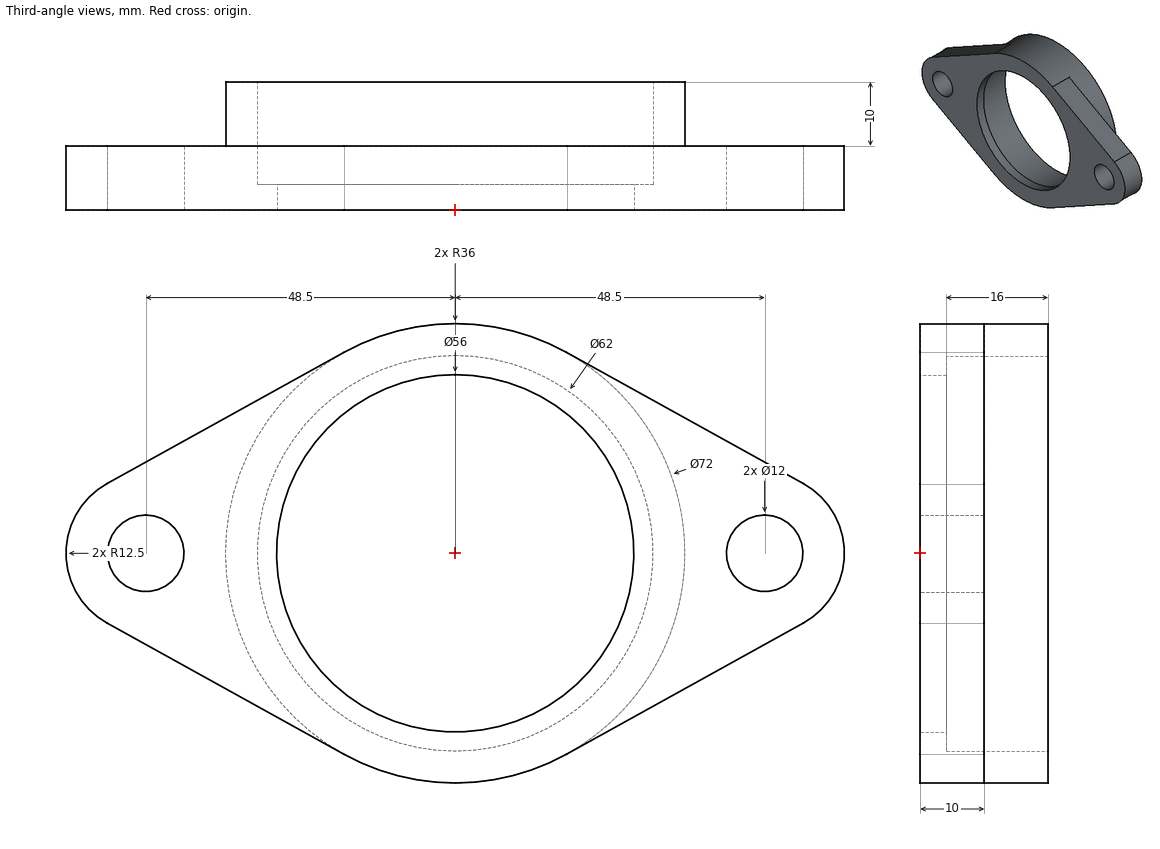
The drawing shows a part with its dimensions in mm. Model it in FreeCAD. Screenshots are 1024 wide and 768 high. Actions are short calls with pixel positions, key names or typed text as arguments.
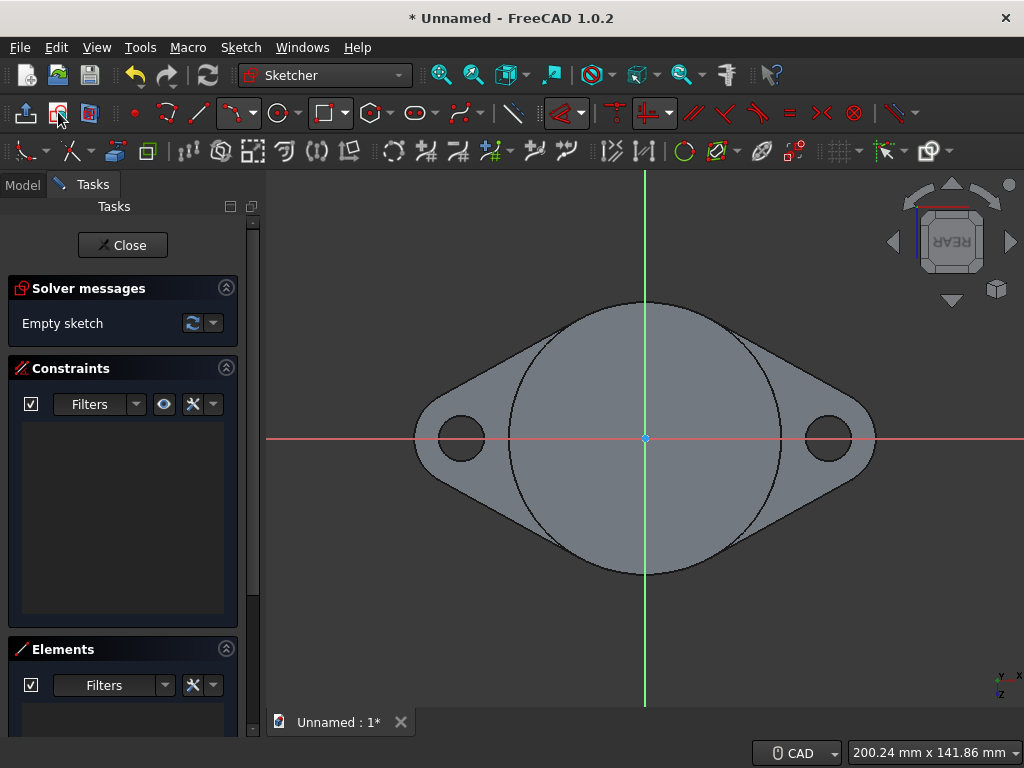
scroll(784, 438, up, 2)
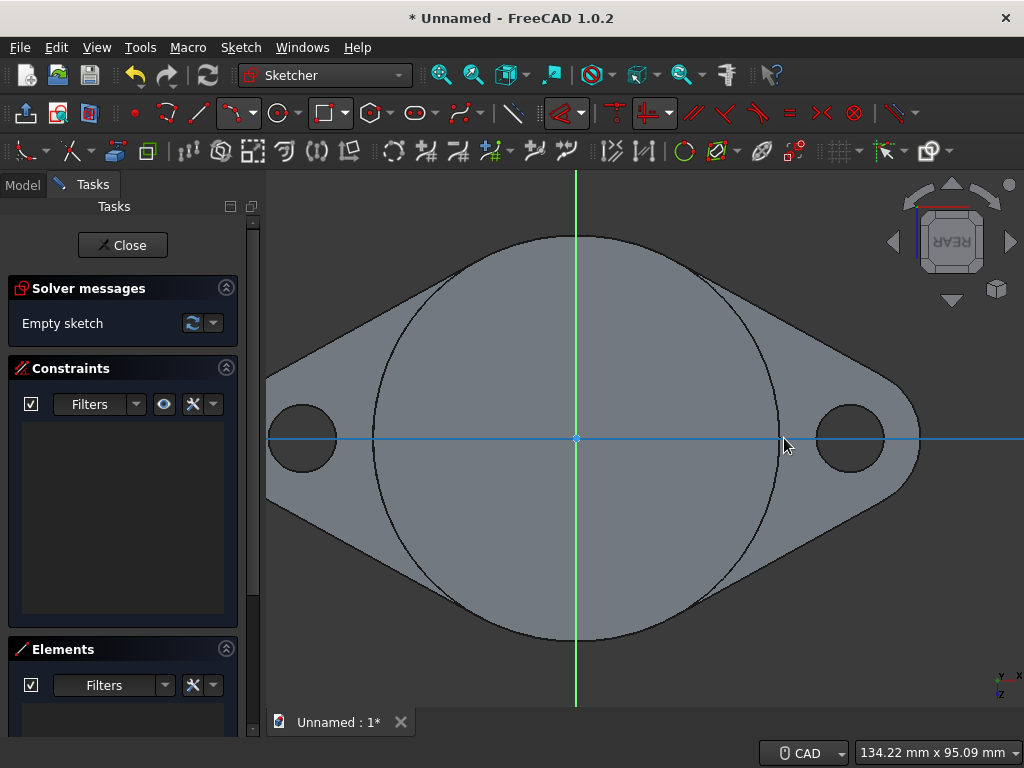
click(278, 114)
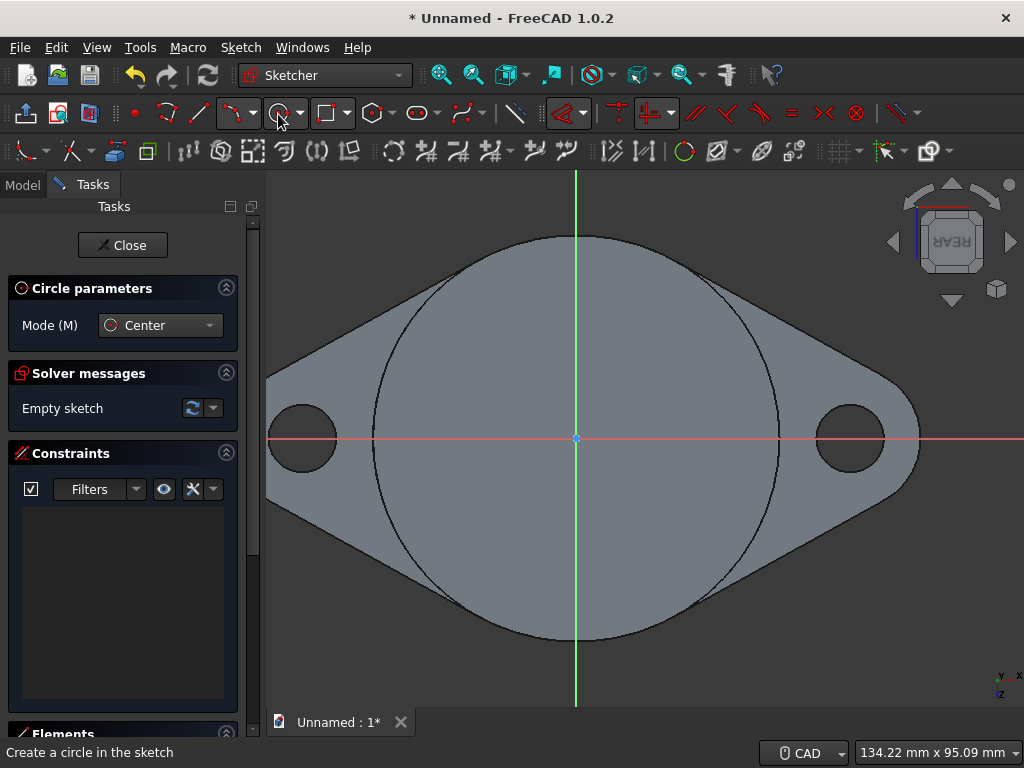
click(576, 438)
click(700, 315)
key(Escape)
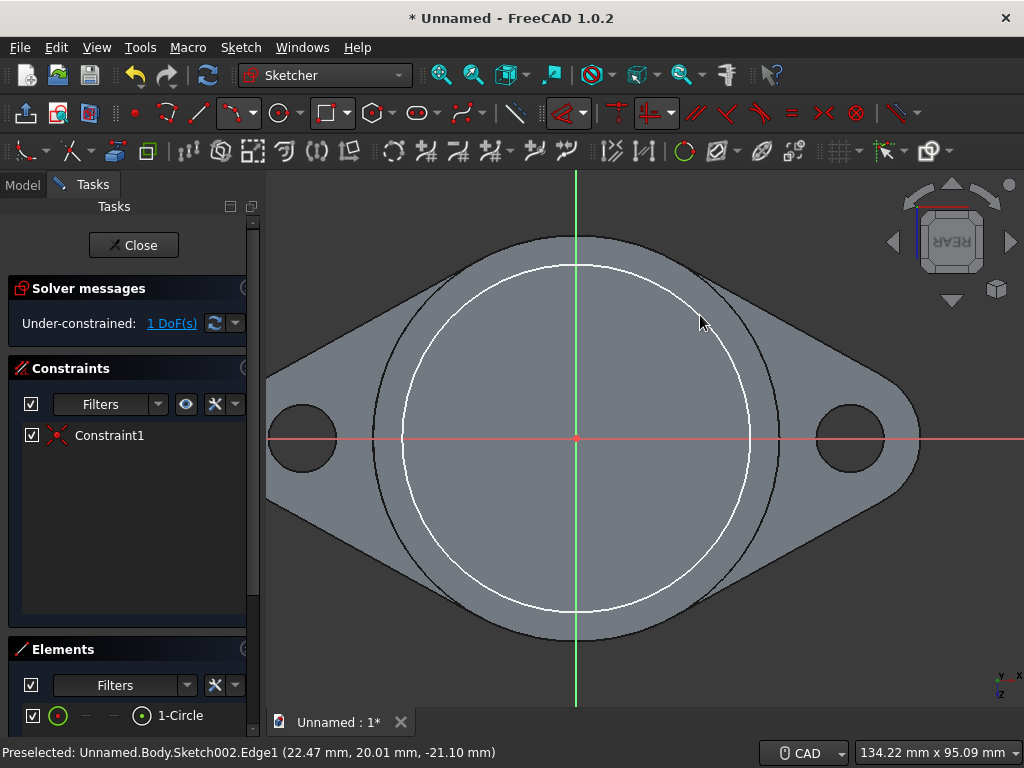
click(699, 315)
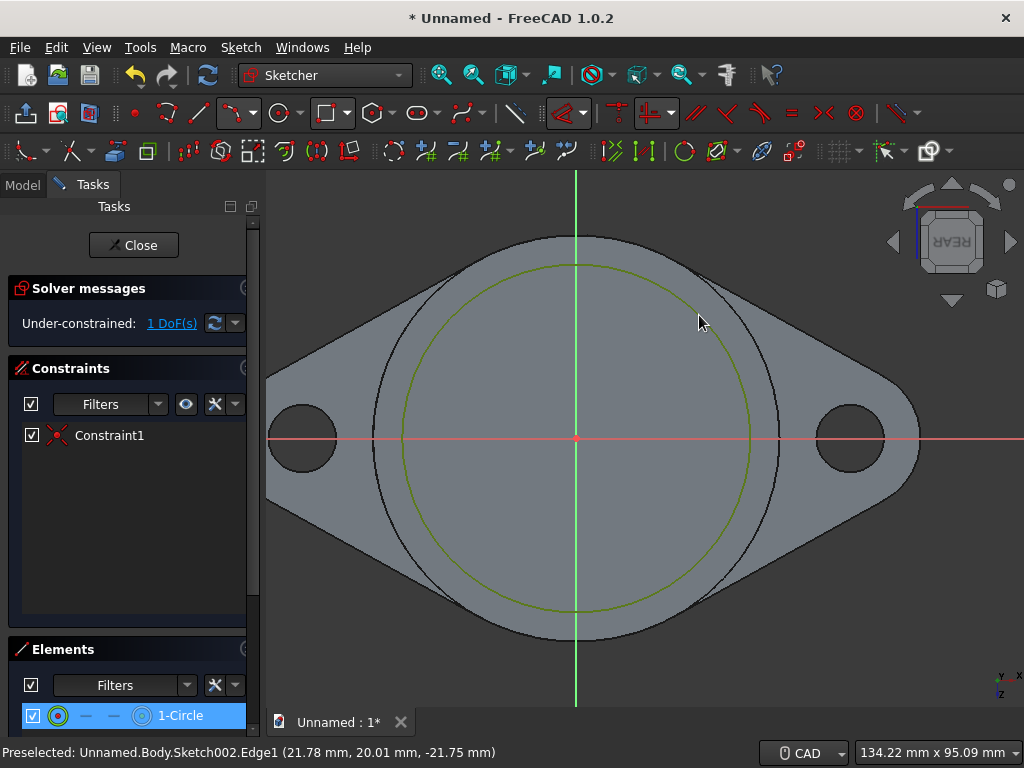
key(k)
key(o)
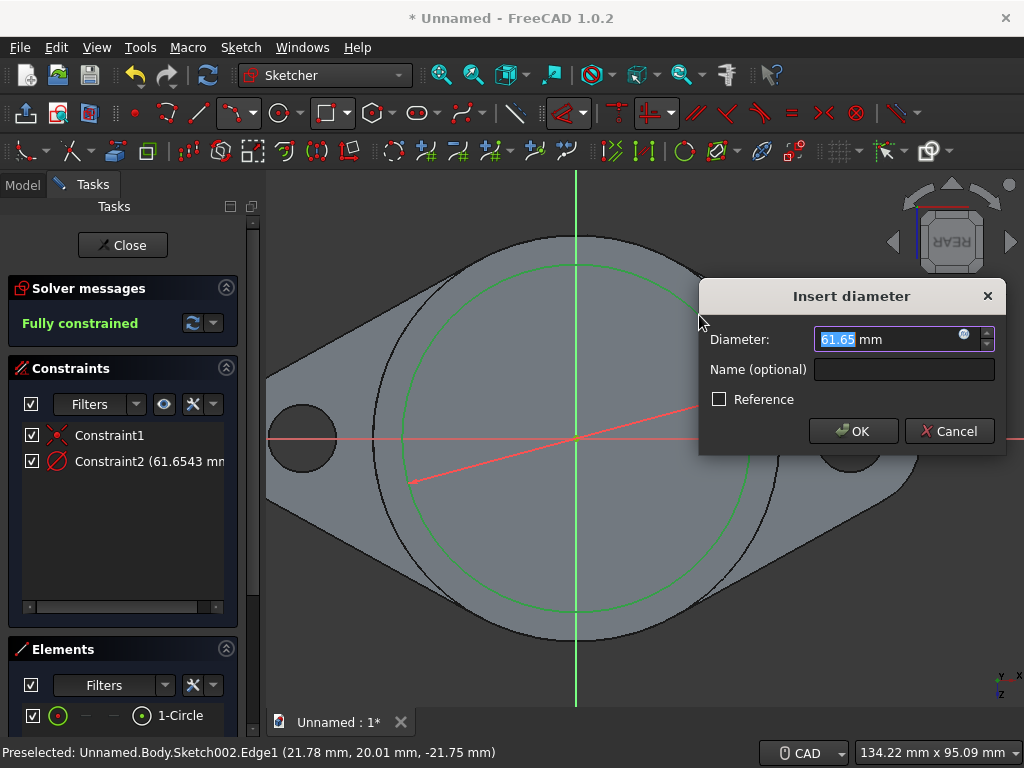
text(62)
key(Return)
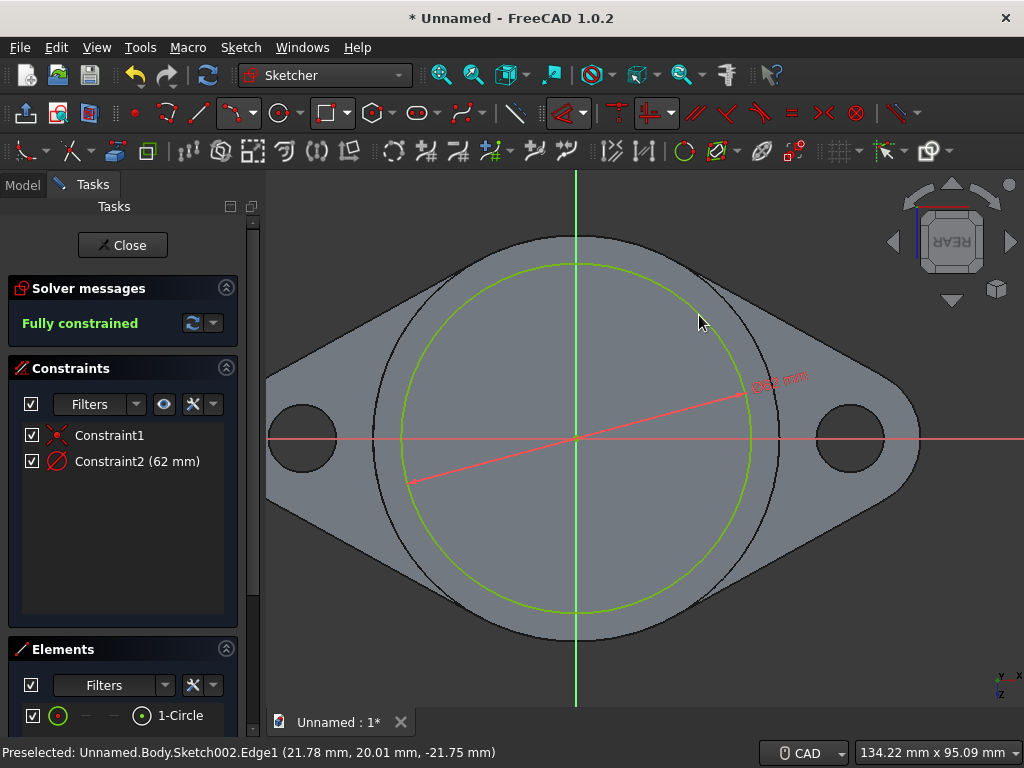
click(123, 245)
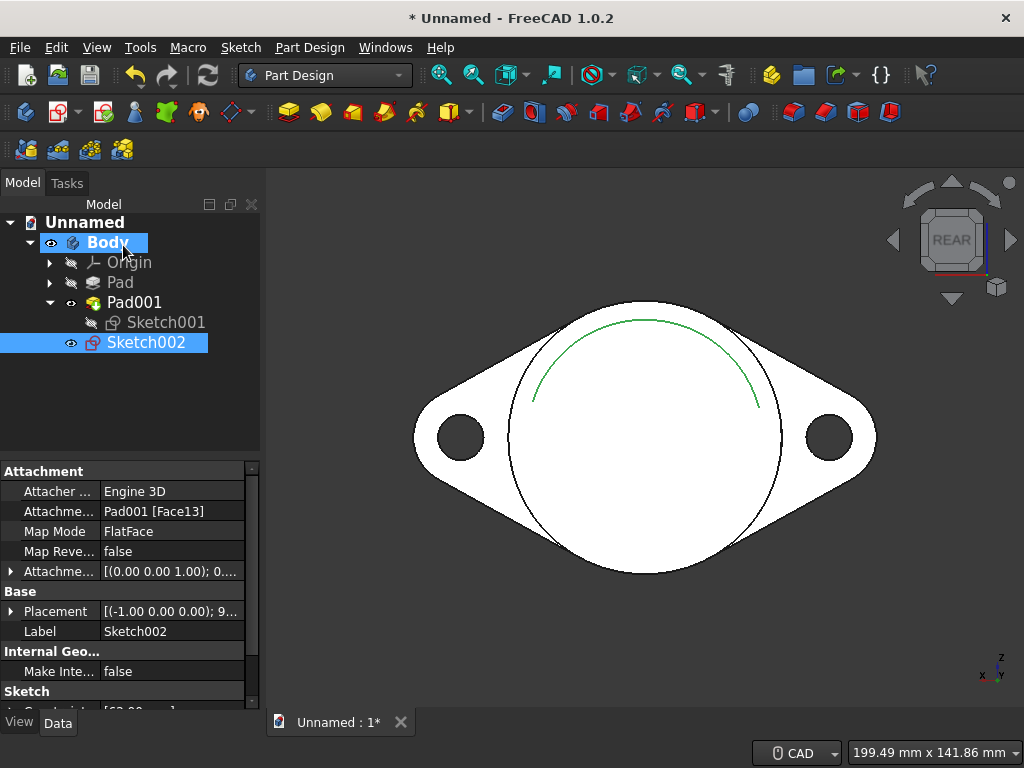
click(504, 112)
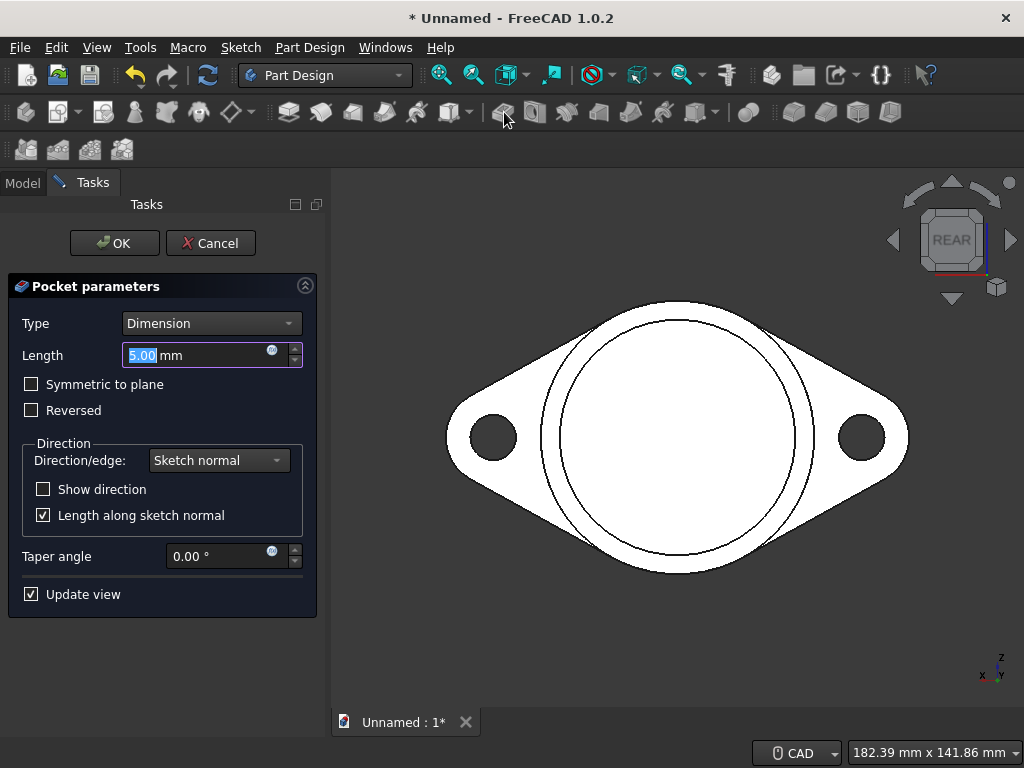
text(16)
key(Tab)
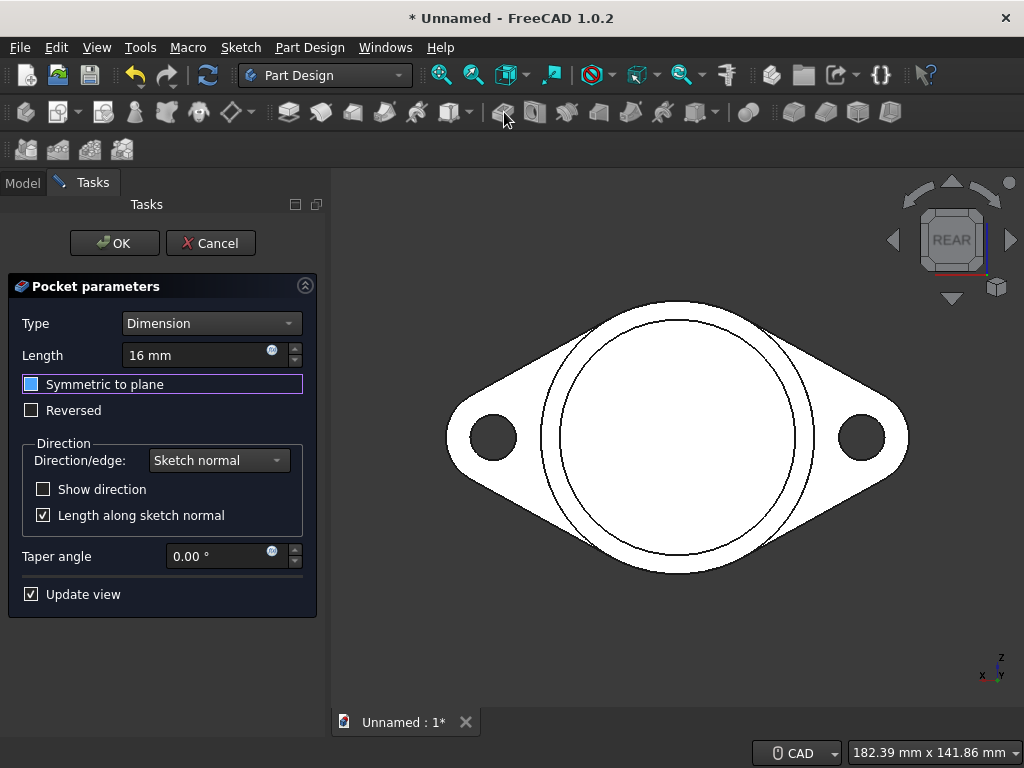
click(115, 243)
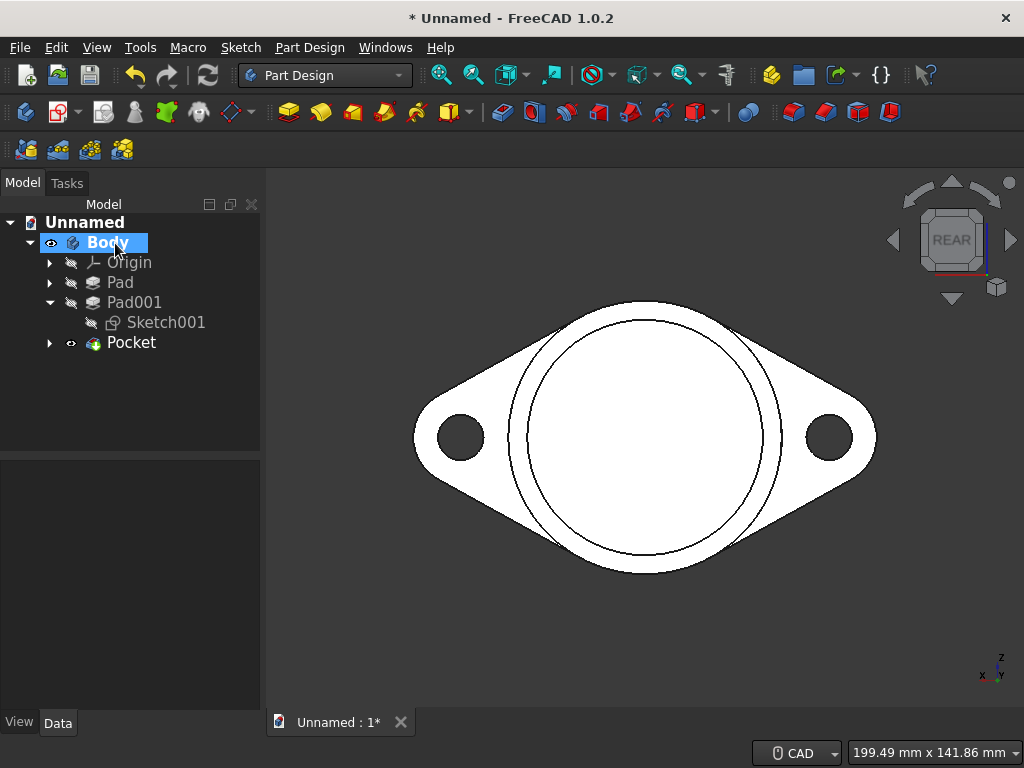
click(645, 437)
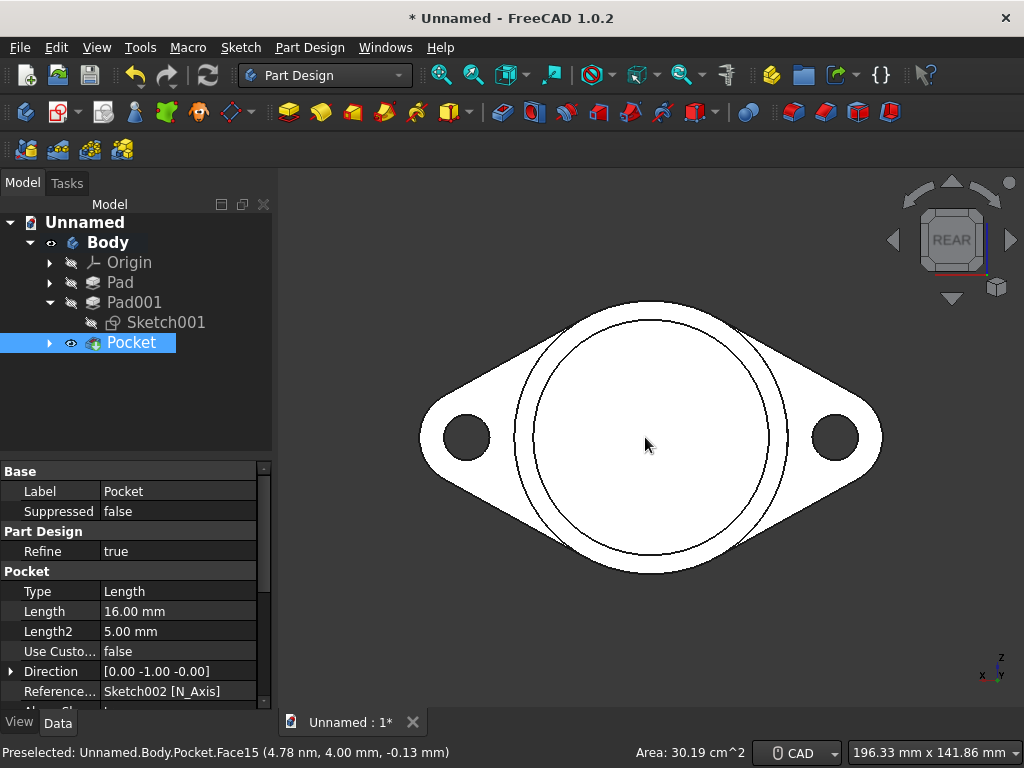
click(58, 112)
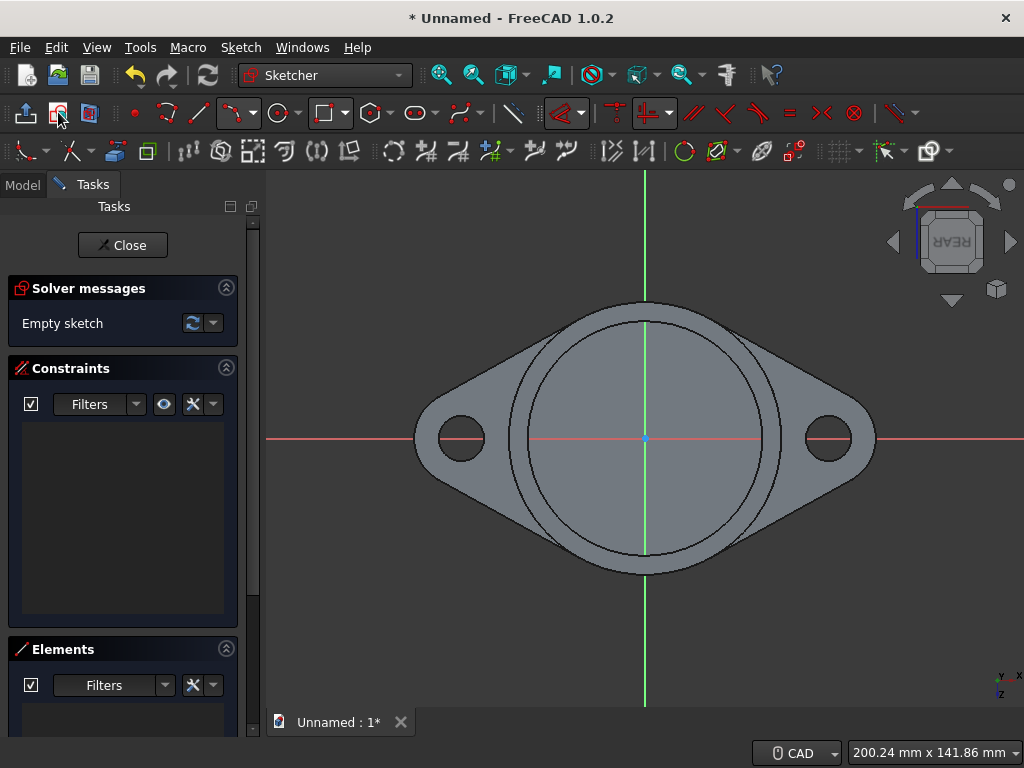
scroll(784, 438, up, 2)